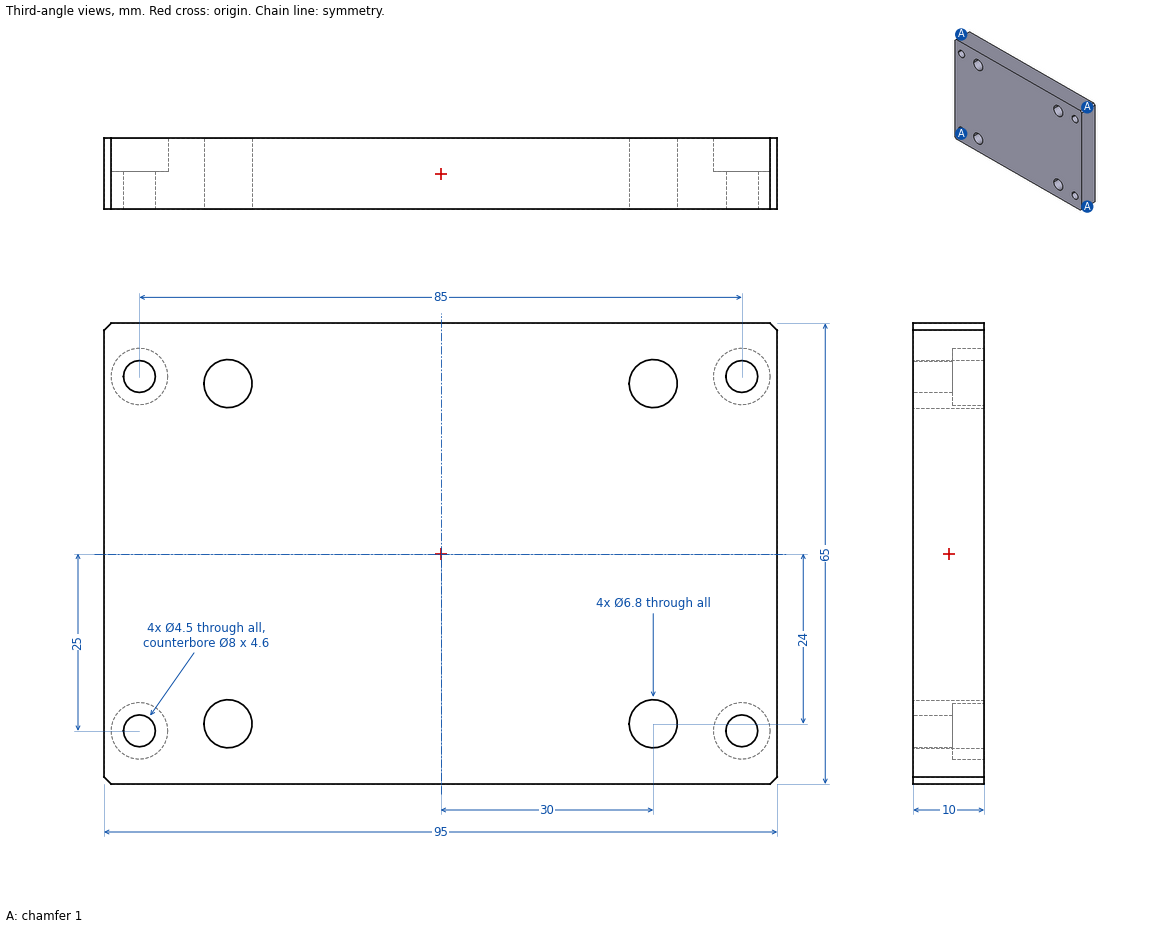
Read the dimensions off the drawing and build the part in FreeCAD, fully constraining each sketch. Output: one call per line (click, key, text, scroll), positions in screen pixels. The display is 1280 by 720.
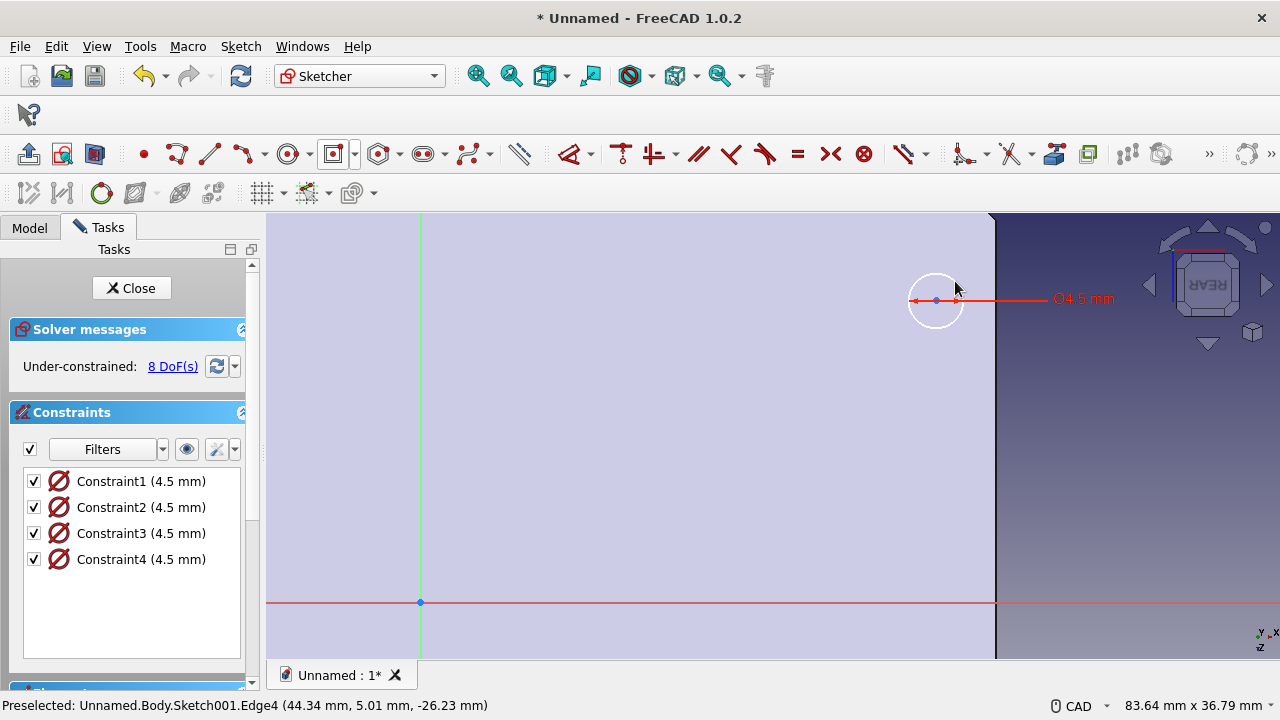
scroll(936, 300, down, 4)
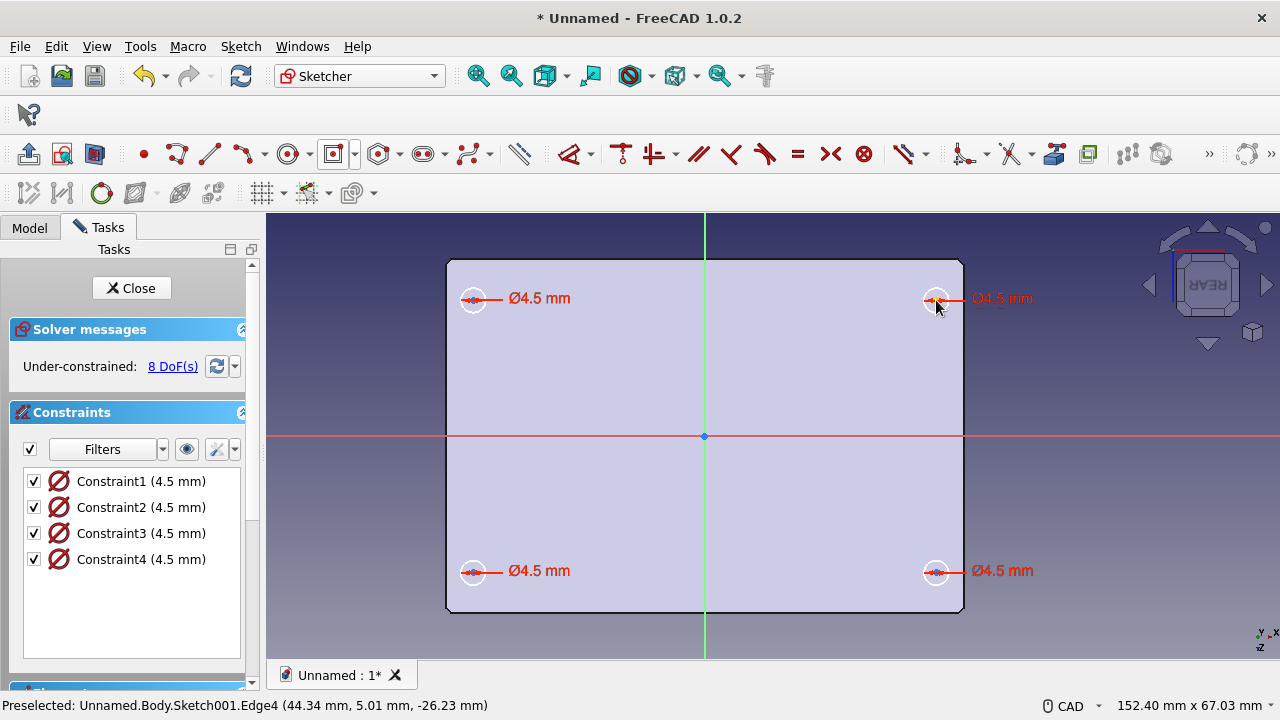
click(473, 300)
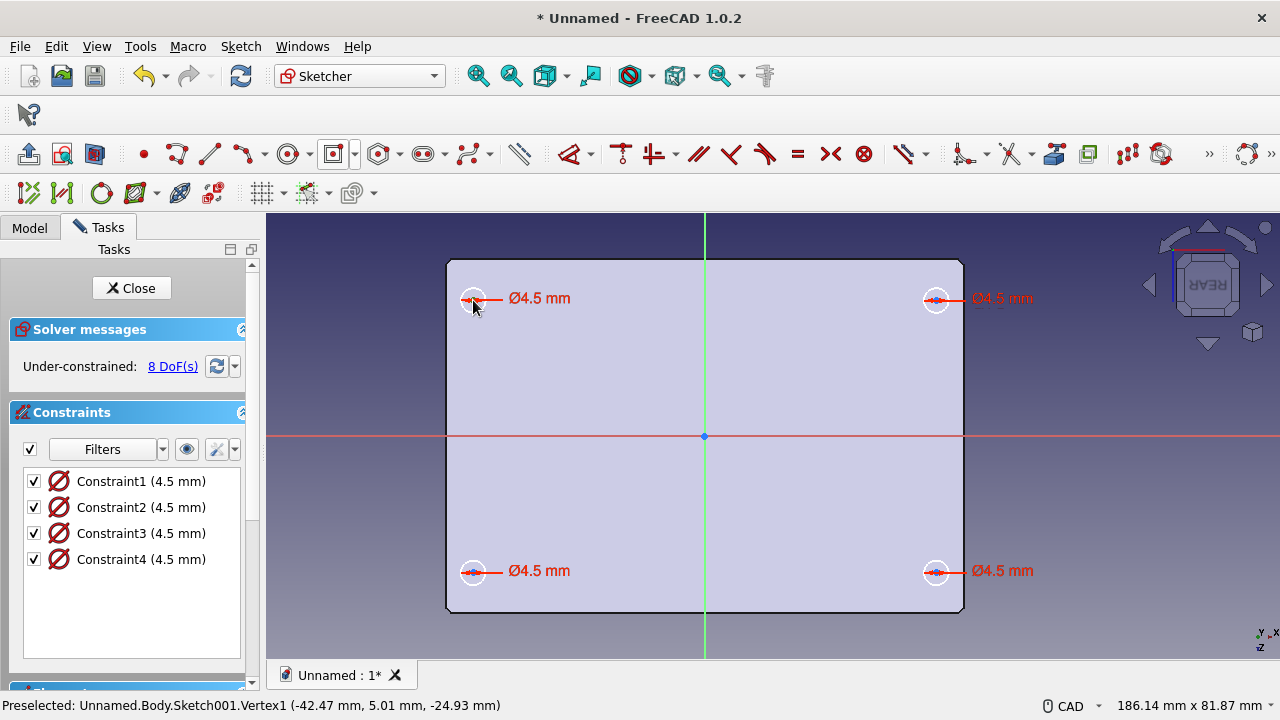
click(473, 573)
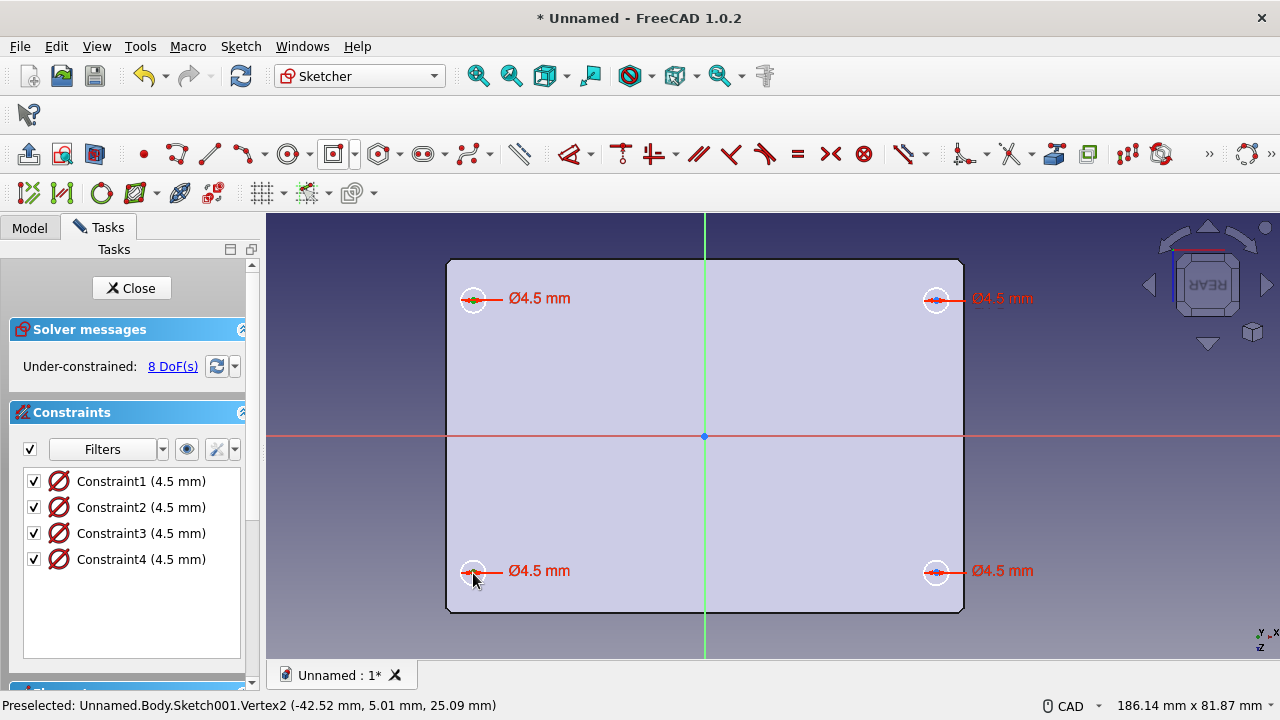
click(353, 436)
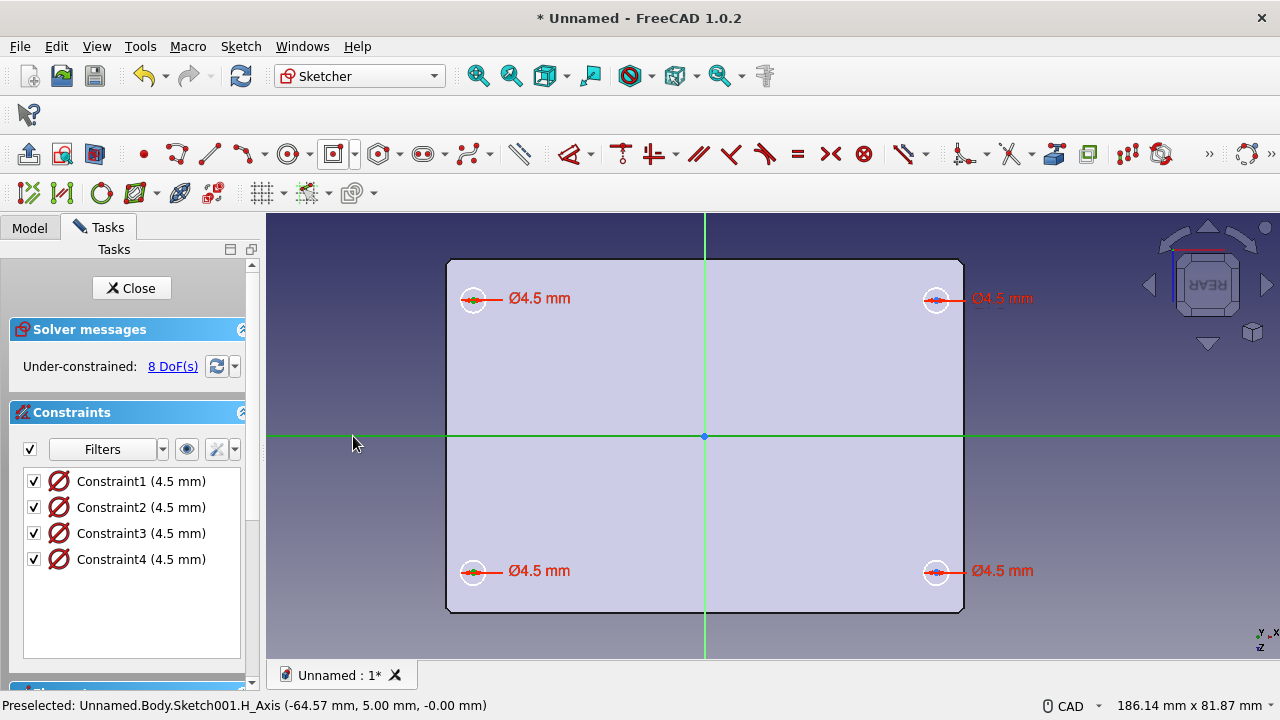
click(831, 154)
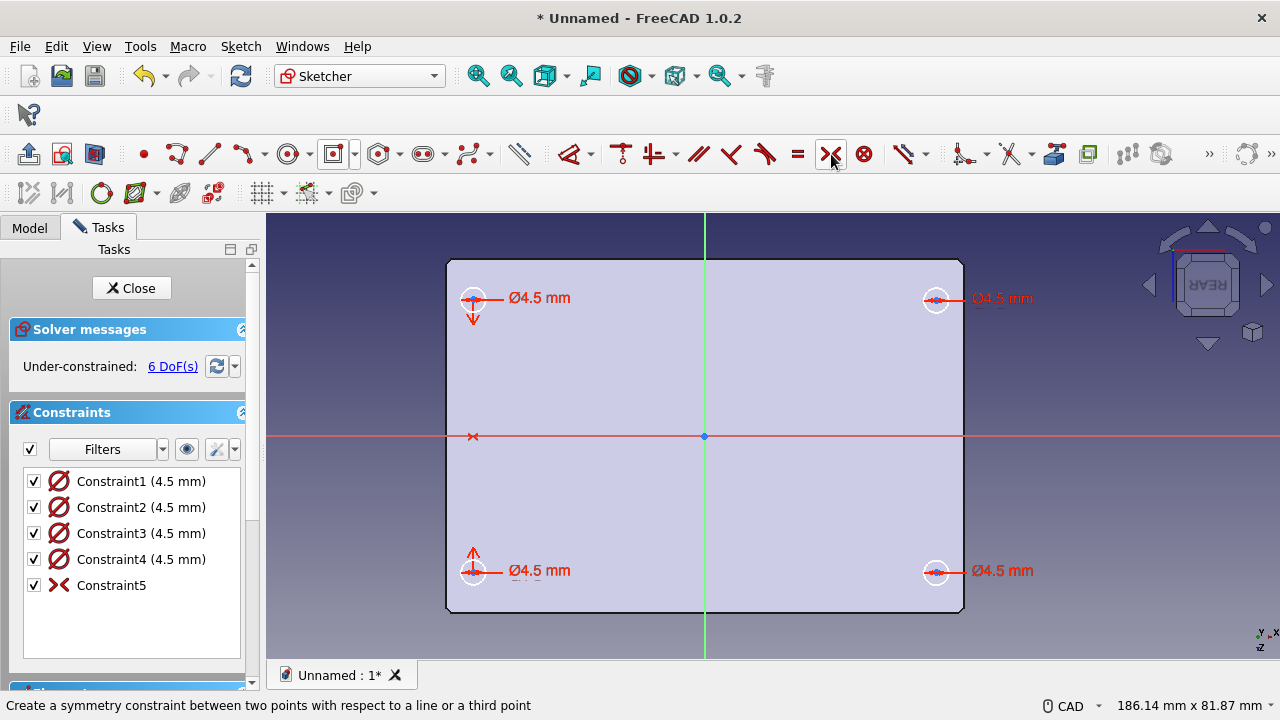
click(473, 573)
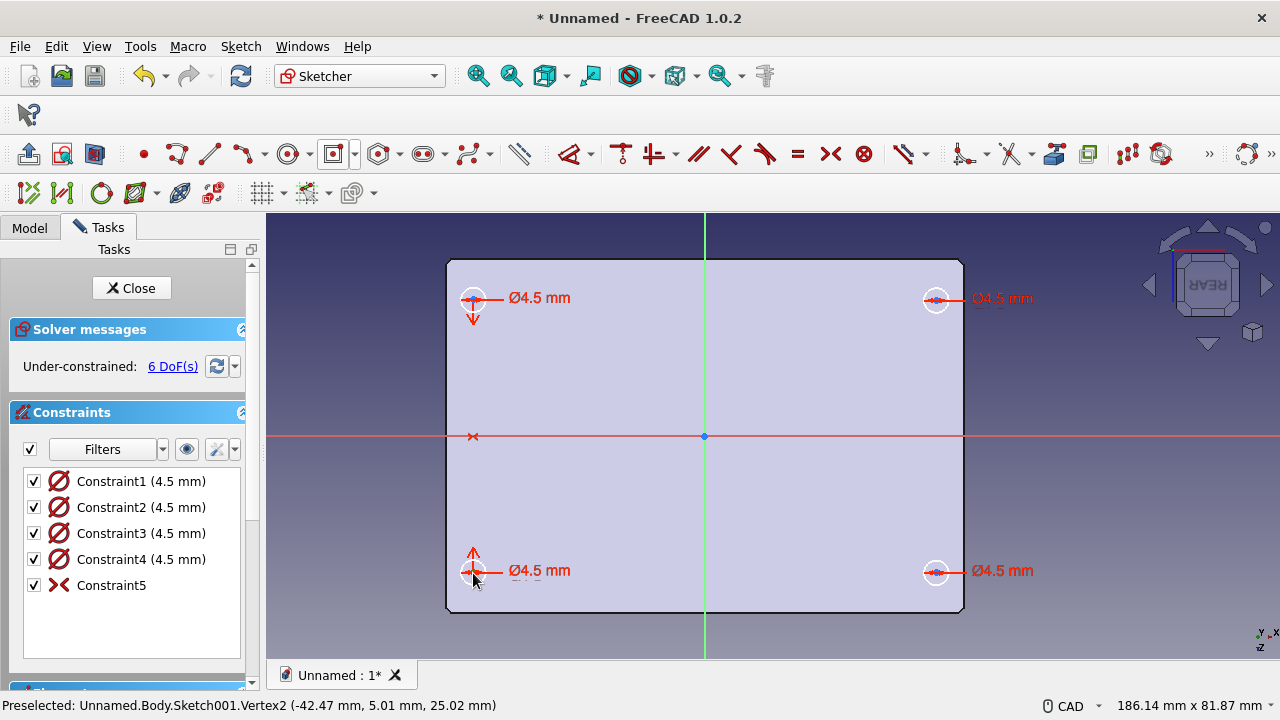
click(936, 573)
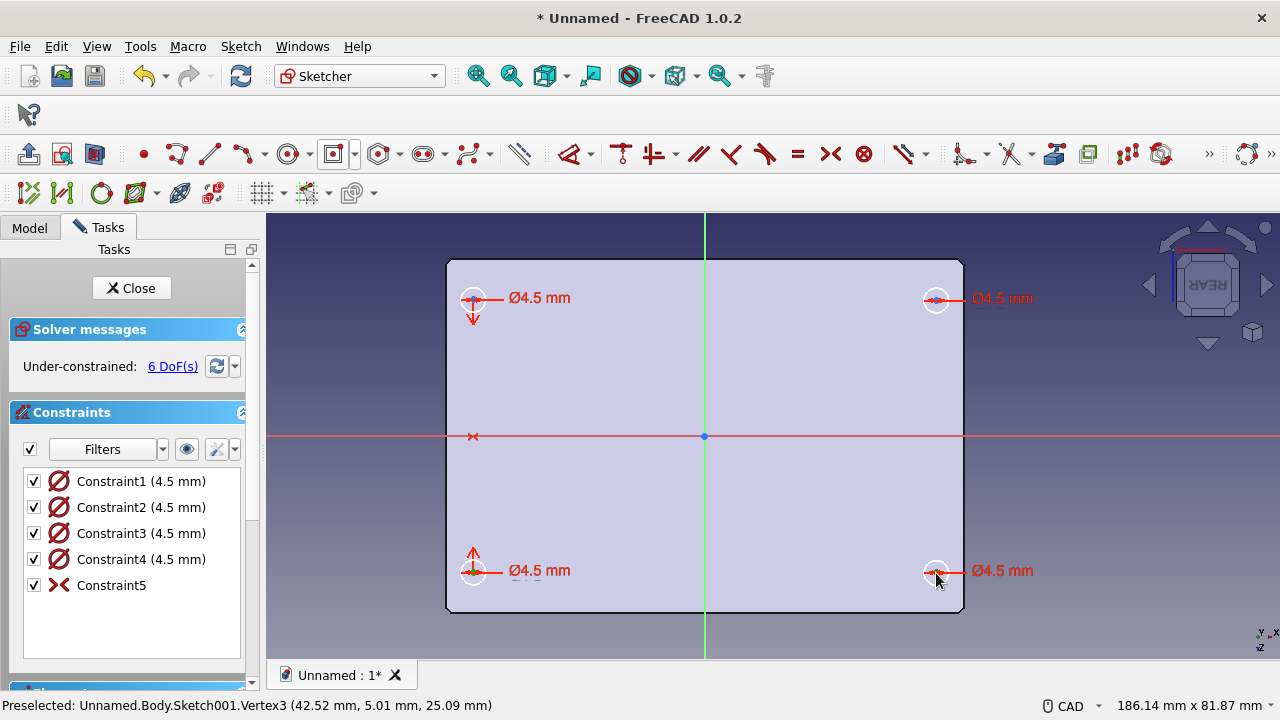
click(705, 603)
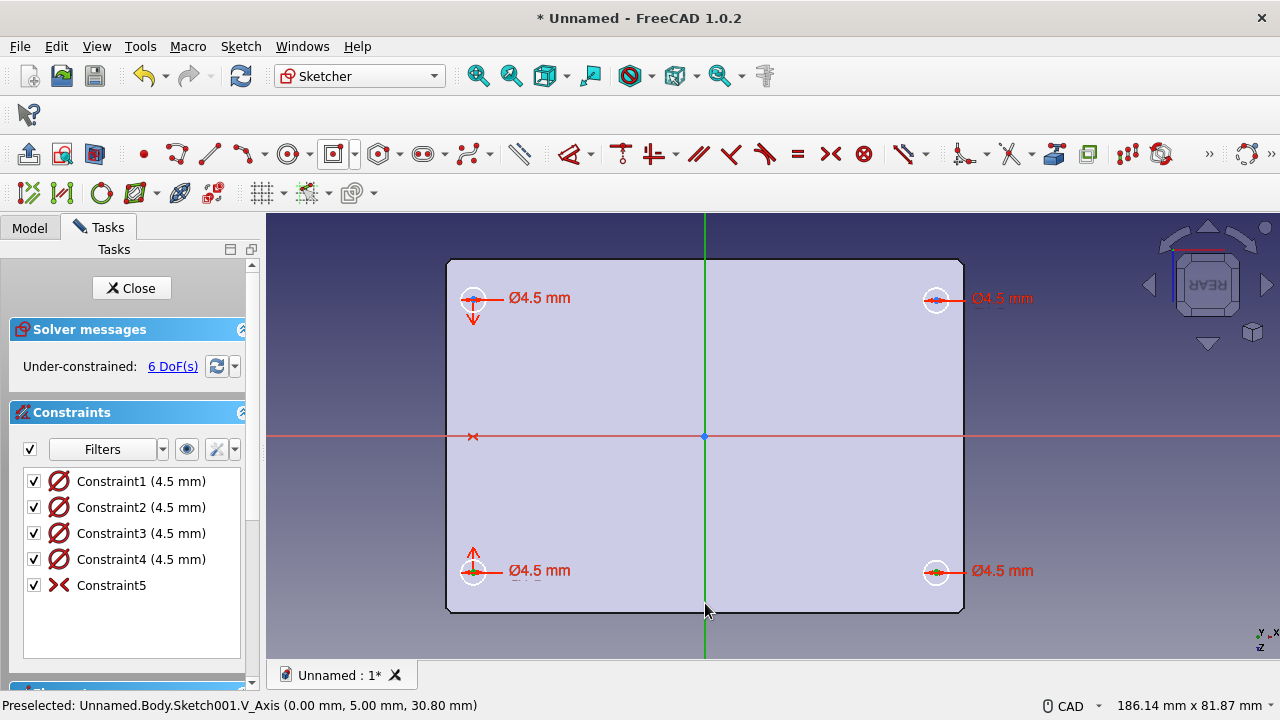
click(831, 154)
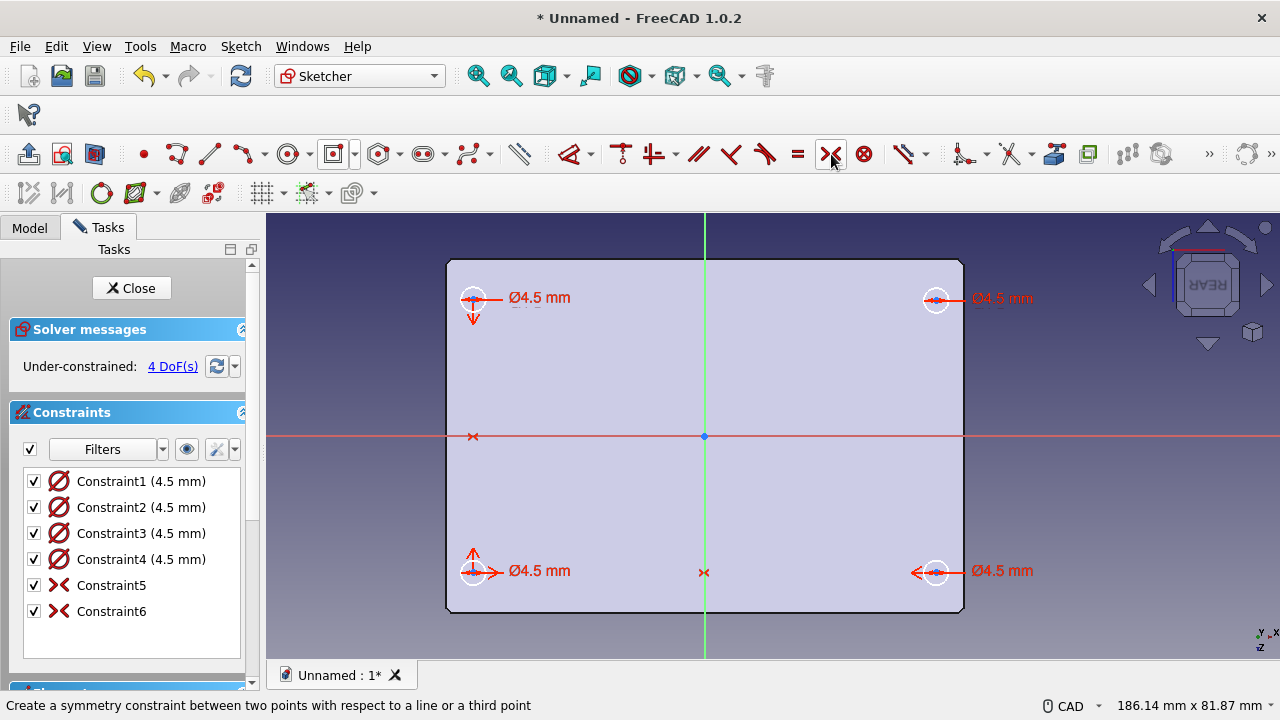
click(473, 300)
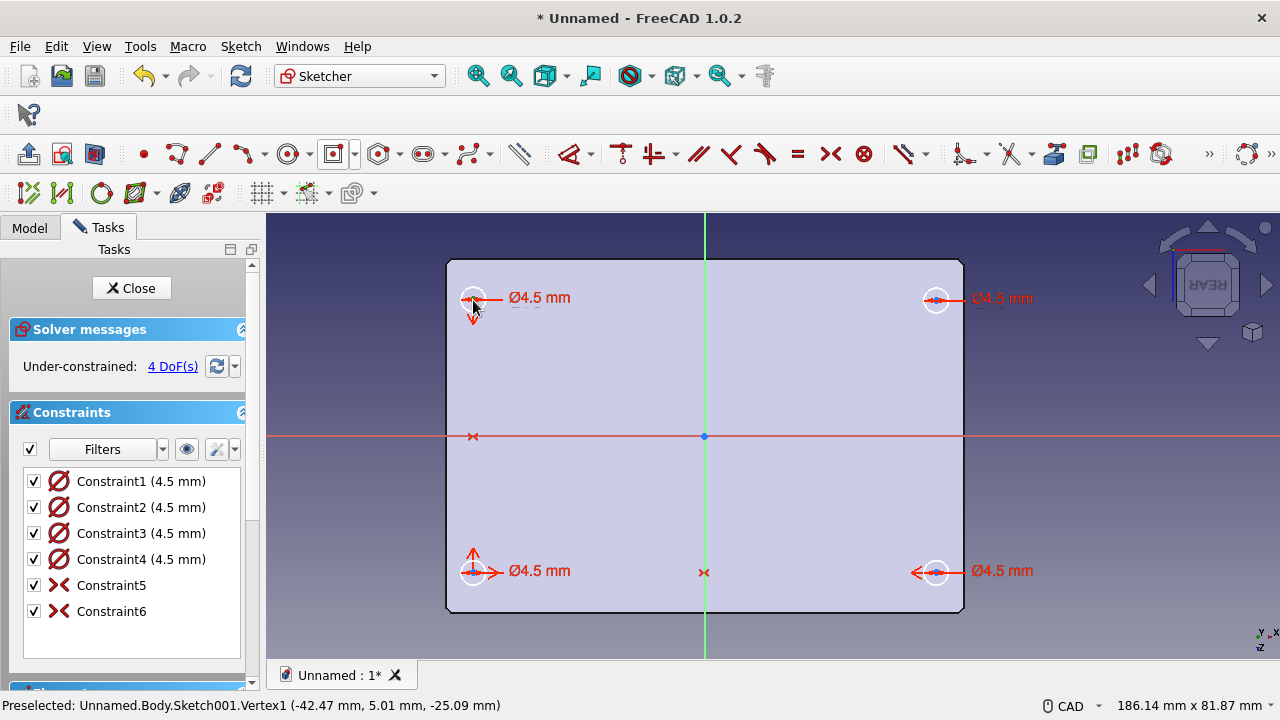
click(936, 301)